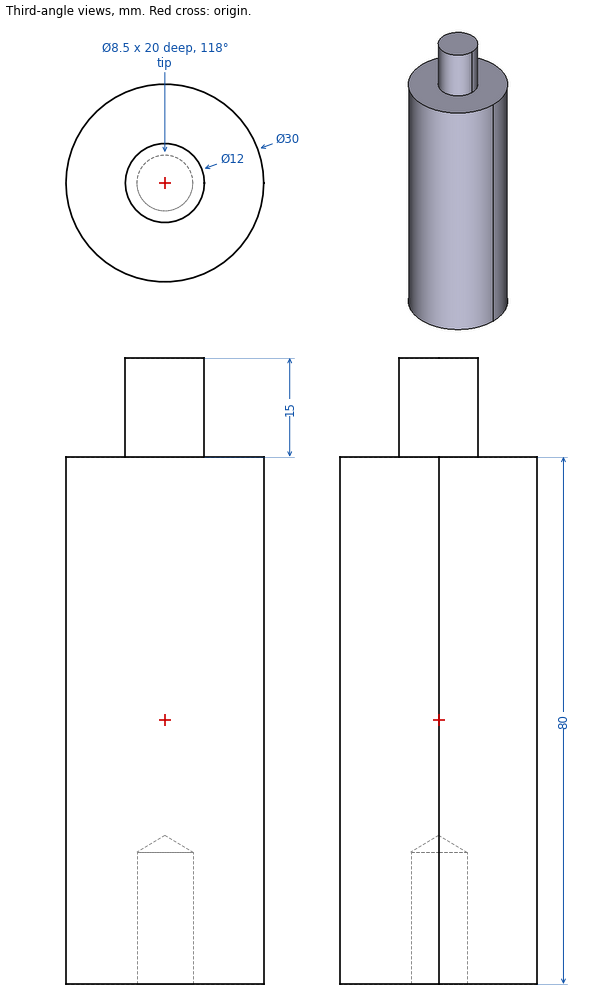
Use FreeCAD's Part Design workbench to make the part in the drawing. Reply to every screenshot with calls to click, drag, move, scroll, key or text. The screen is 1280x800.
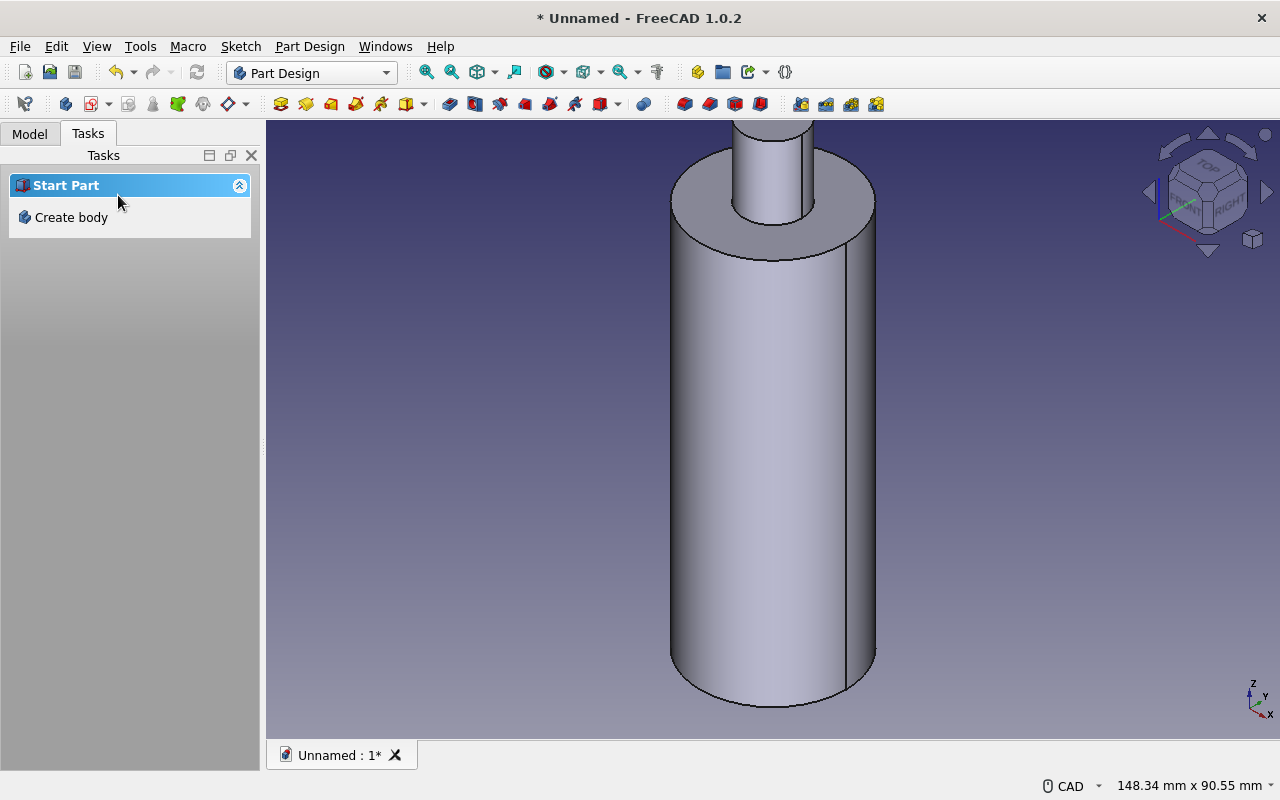
click(427, 72)